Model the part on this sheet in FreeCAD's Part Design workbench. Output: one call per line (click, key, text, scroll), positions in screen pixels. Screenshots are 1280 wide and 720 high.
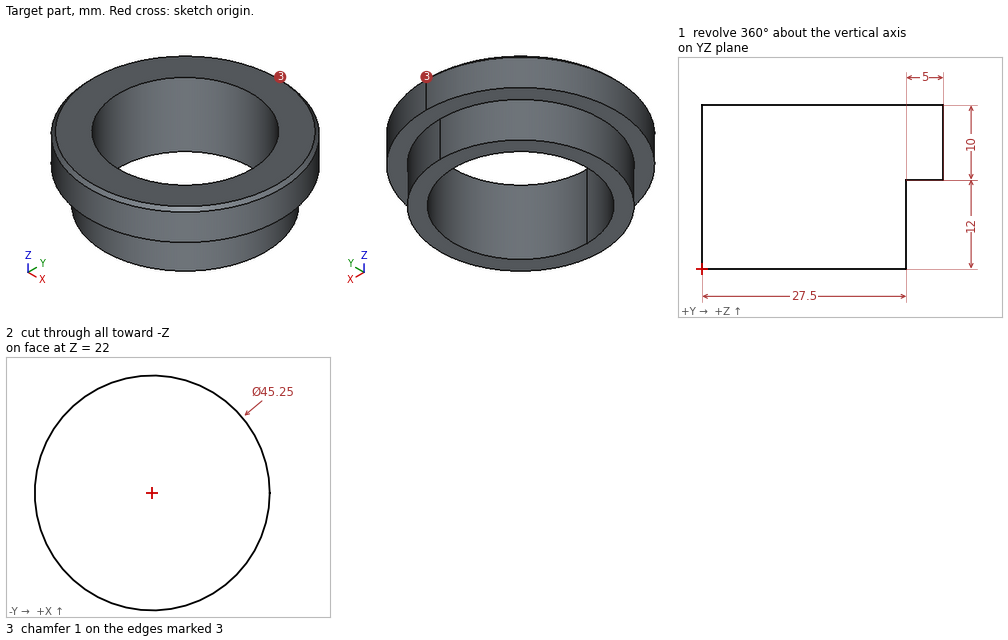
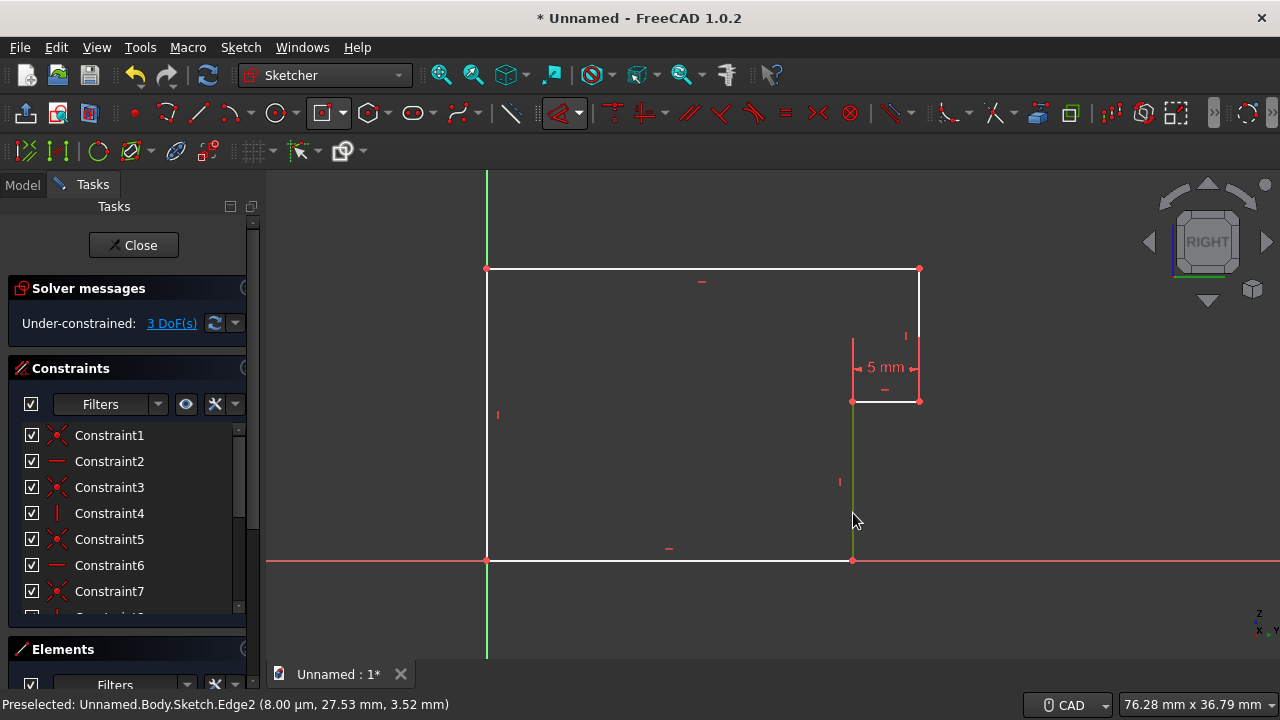
key(i)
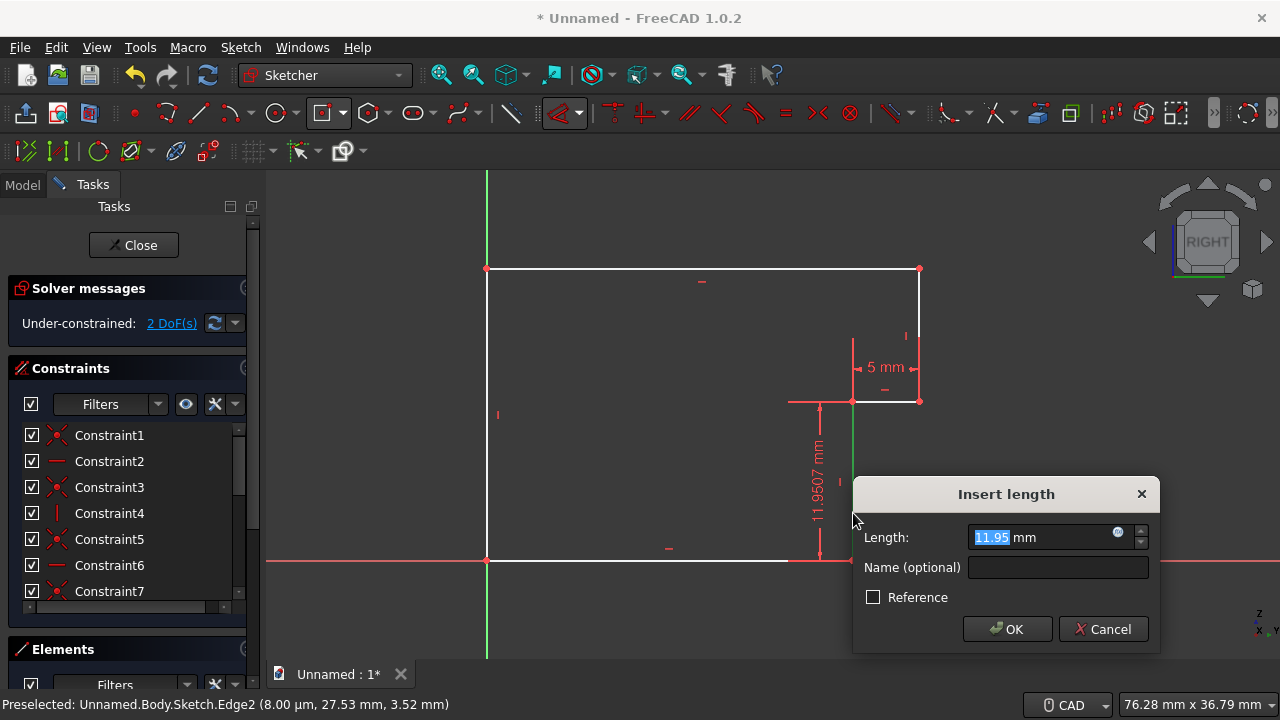
text(12)
key(Return)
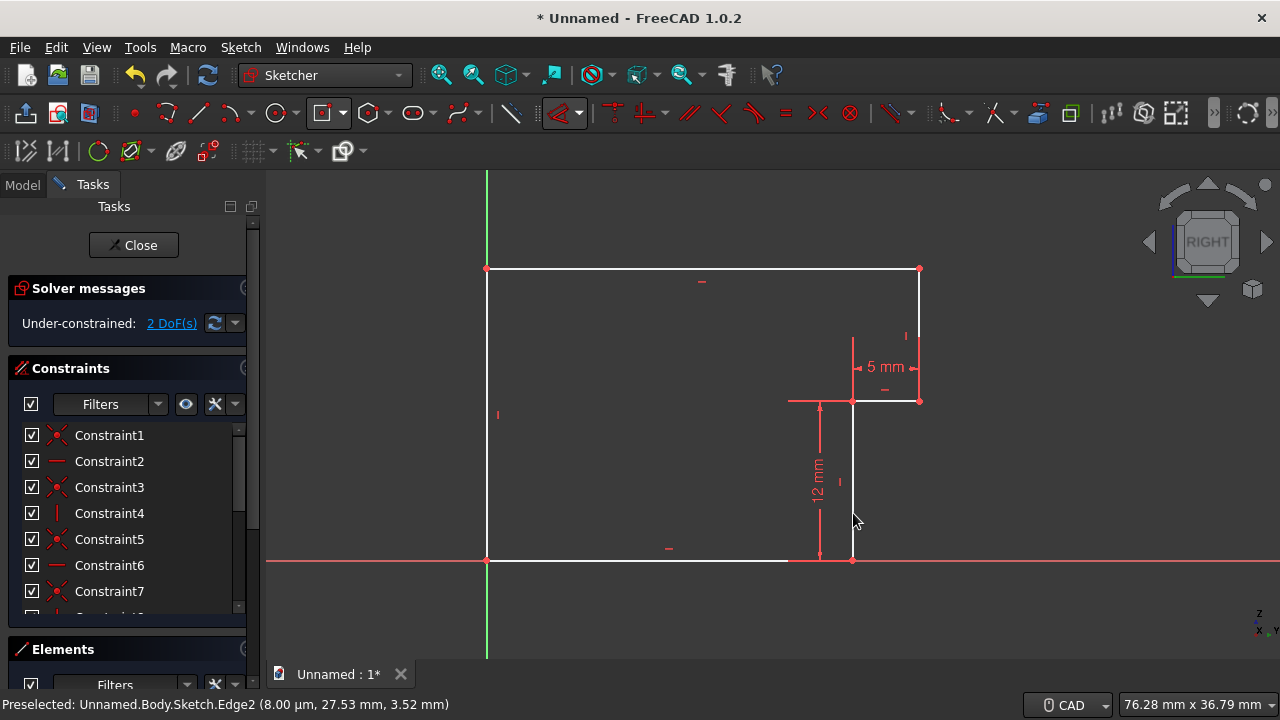
click(919, 362)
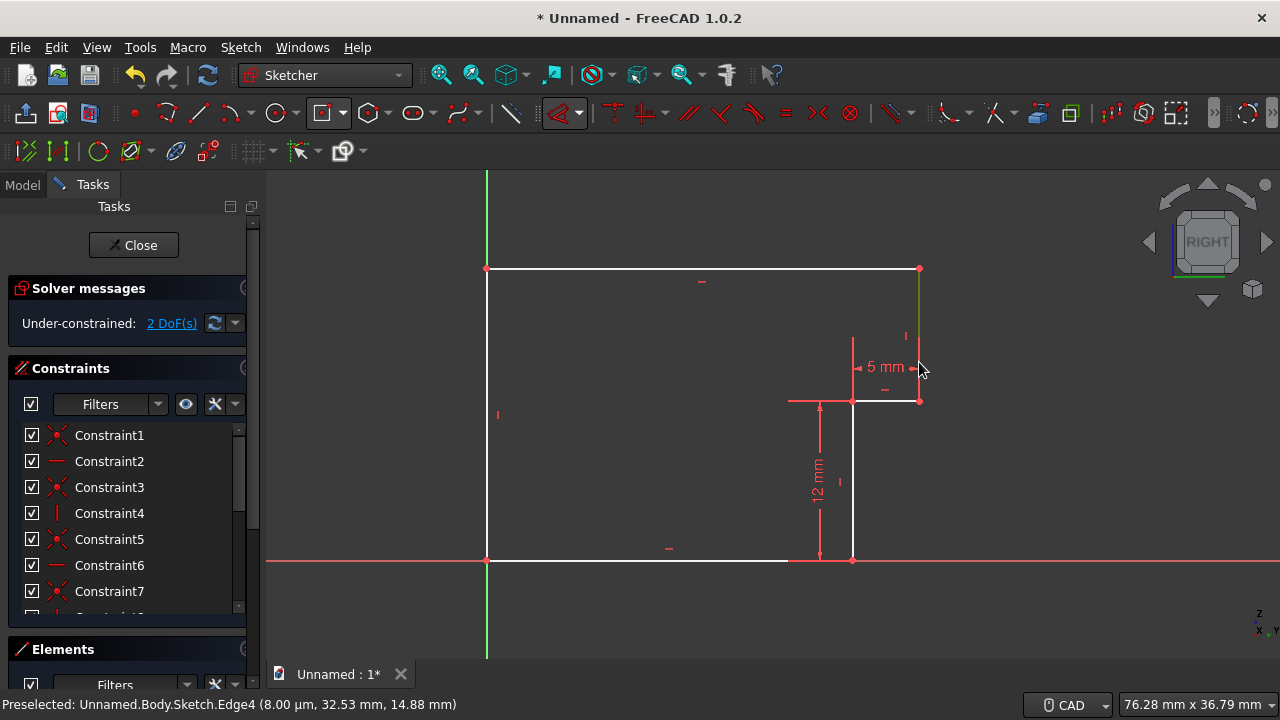
click(582, 114)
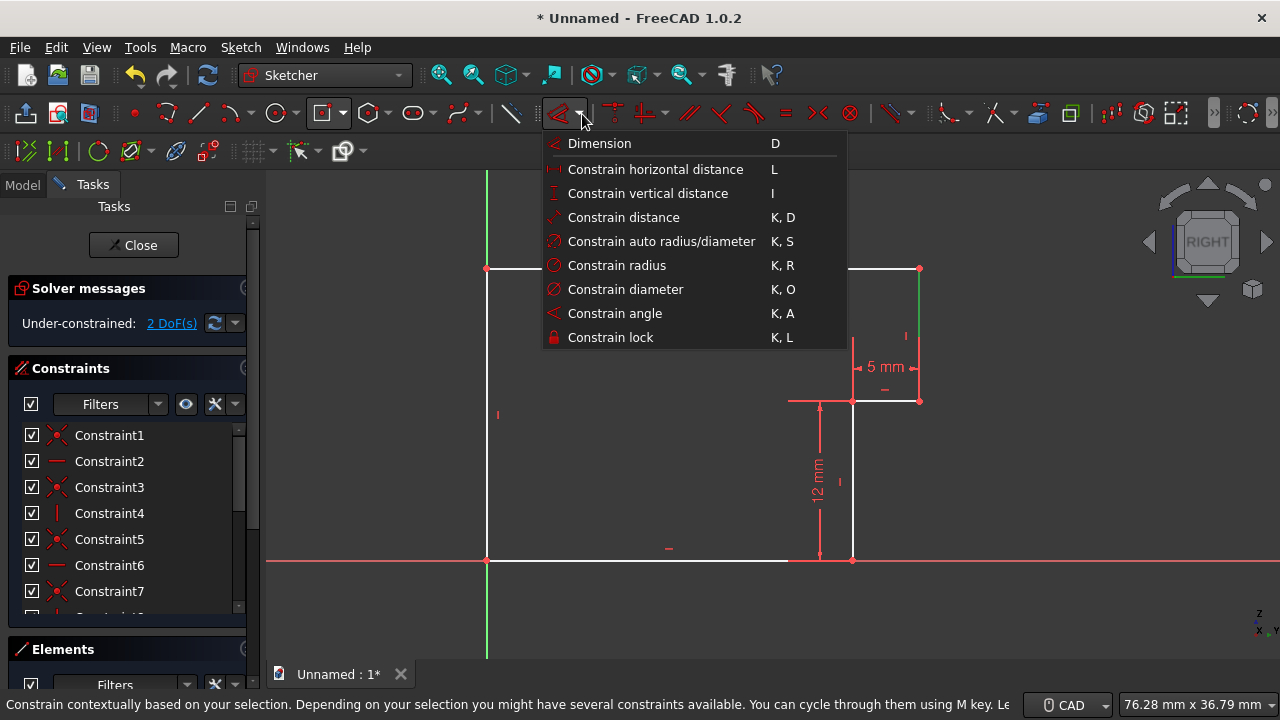
click(695, 193)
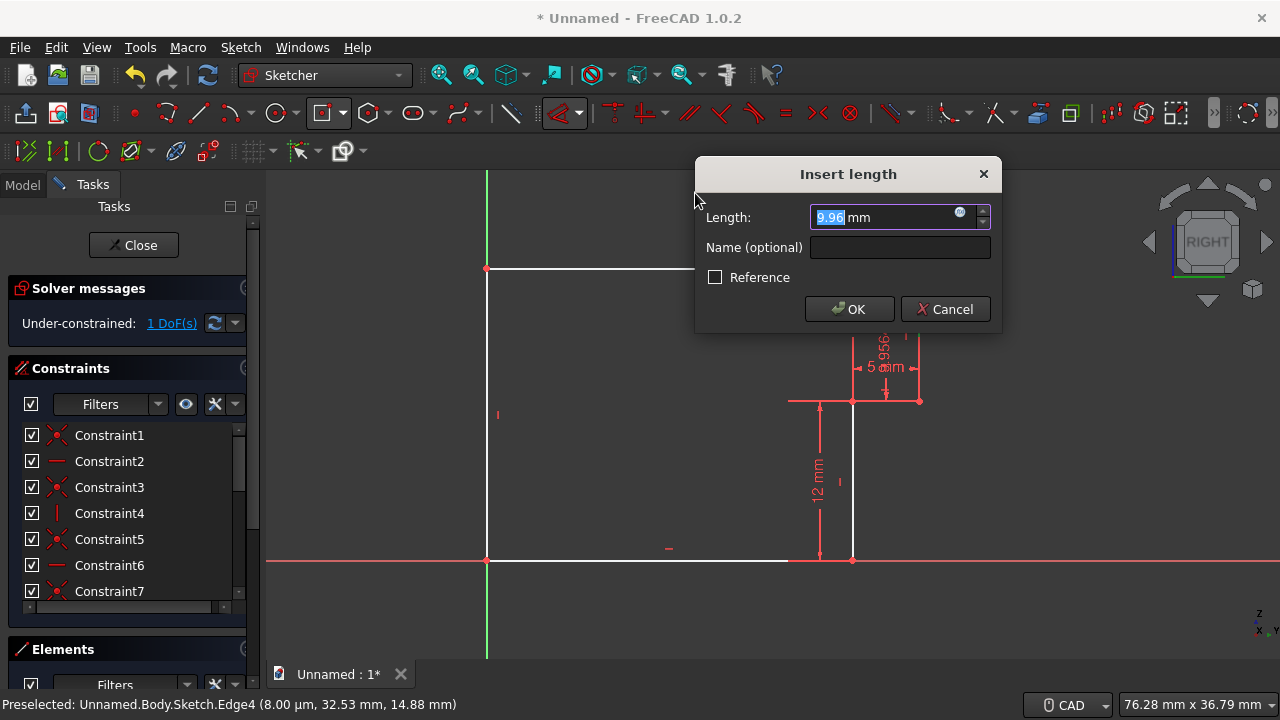
text(10)
key(Return)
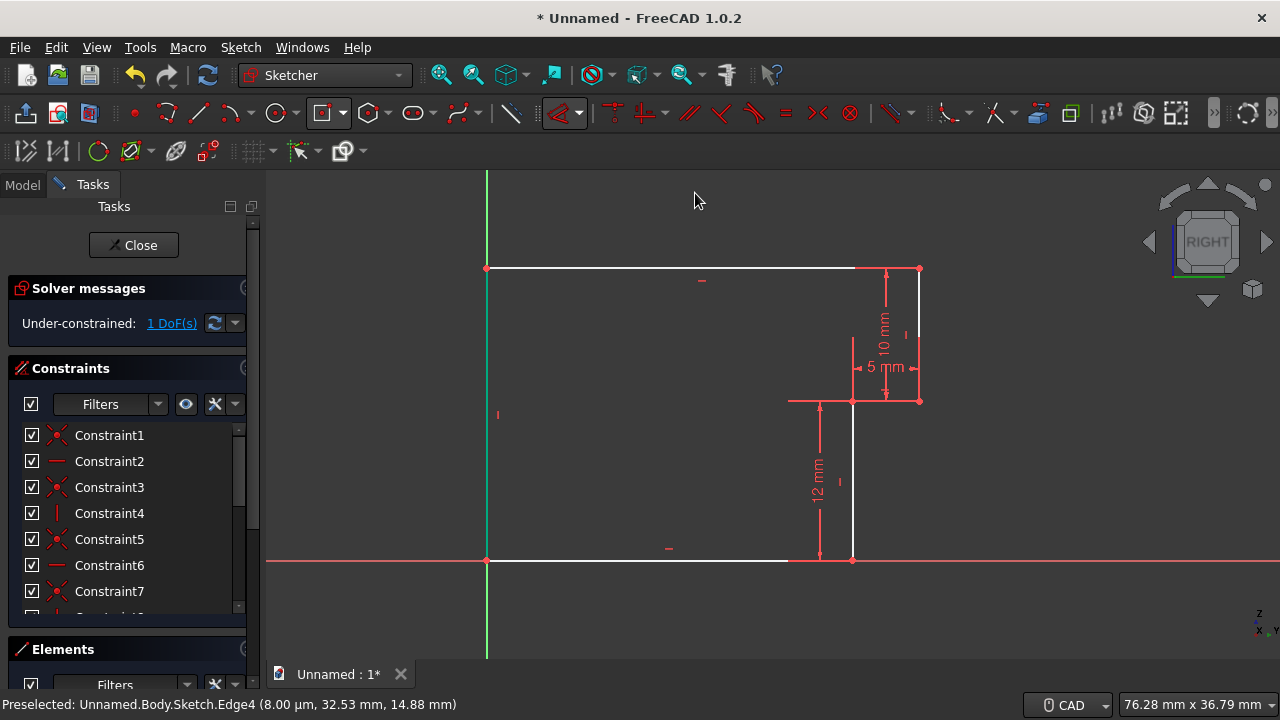
click(596, 561)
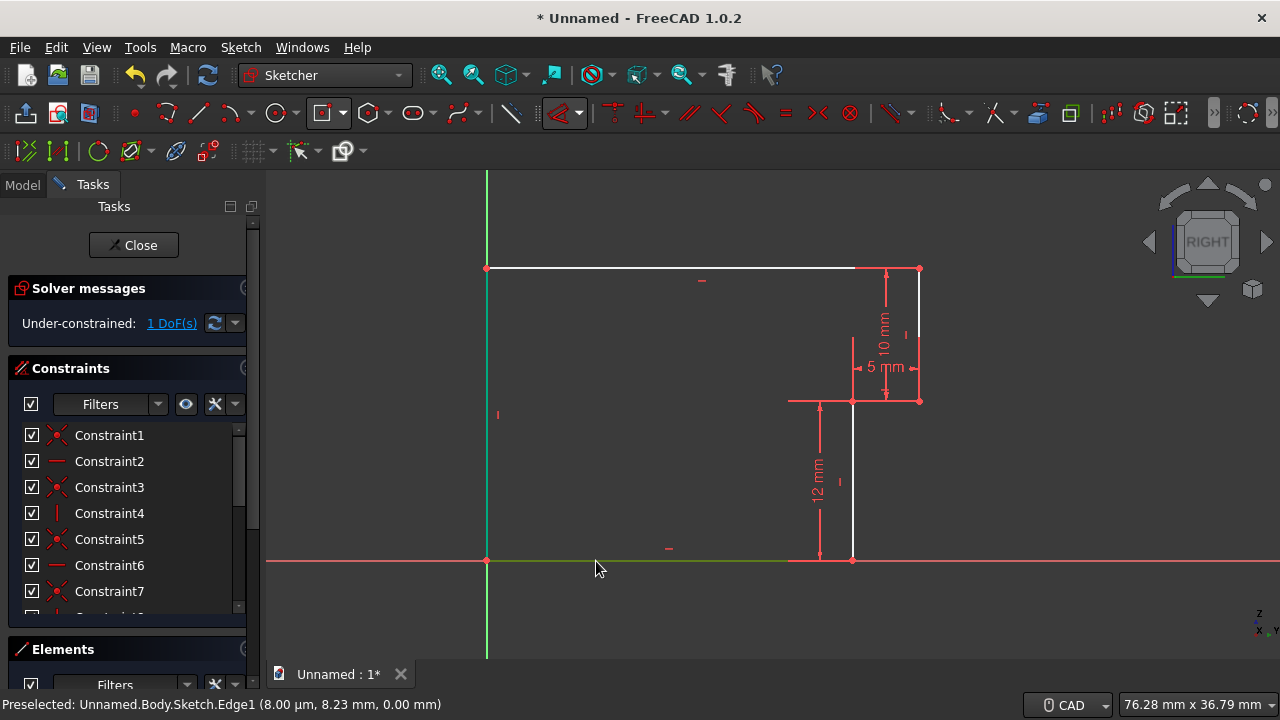
key(l)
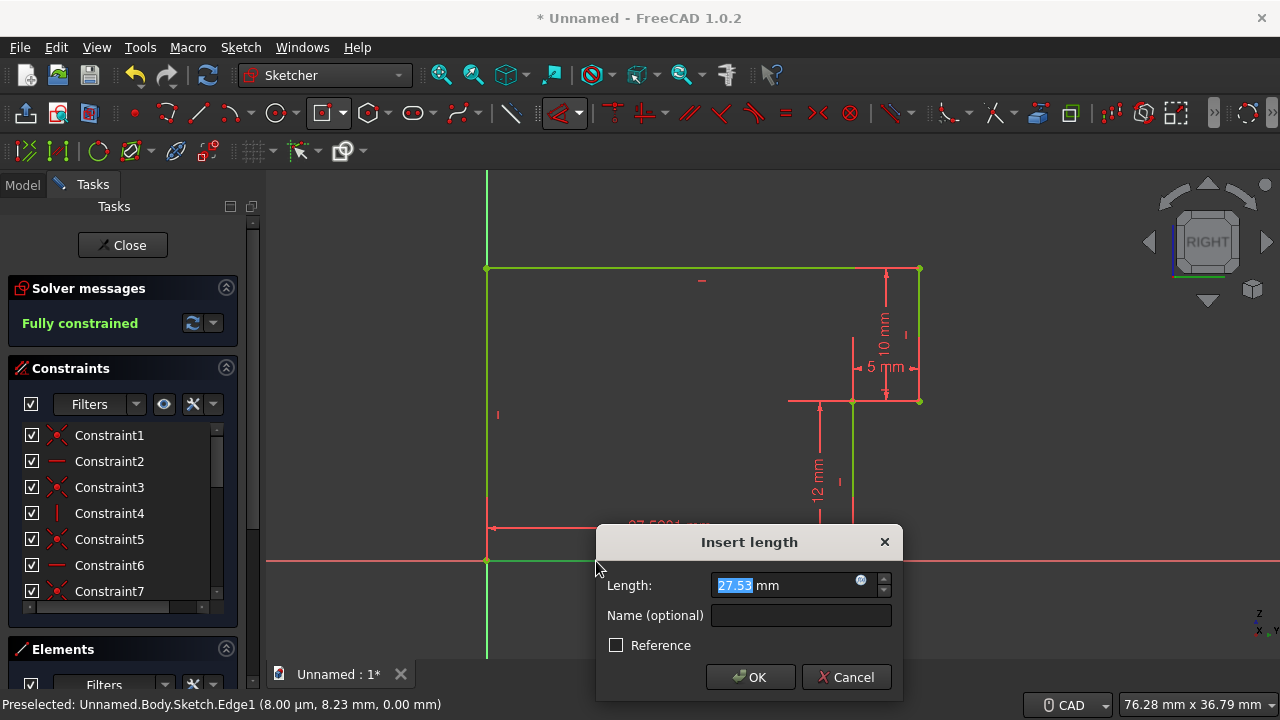
text(27.5)
key(Return)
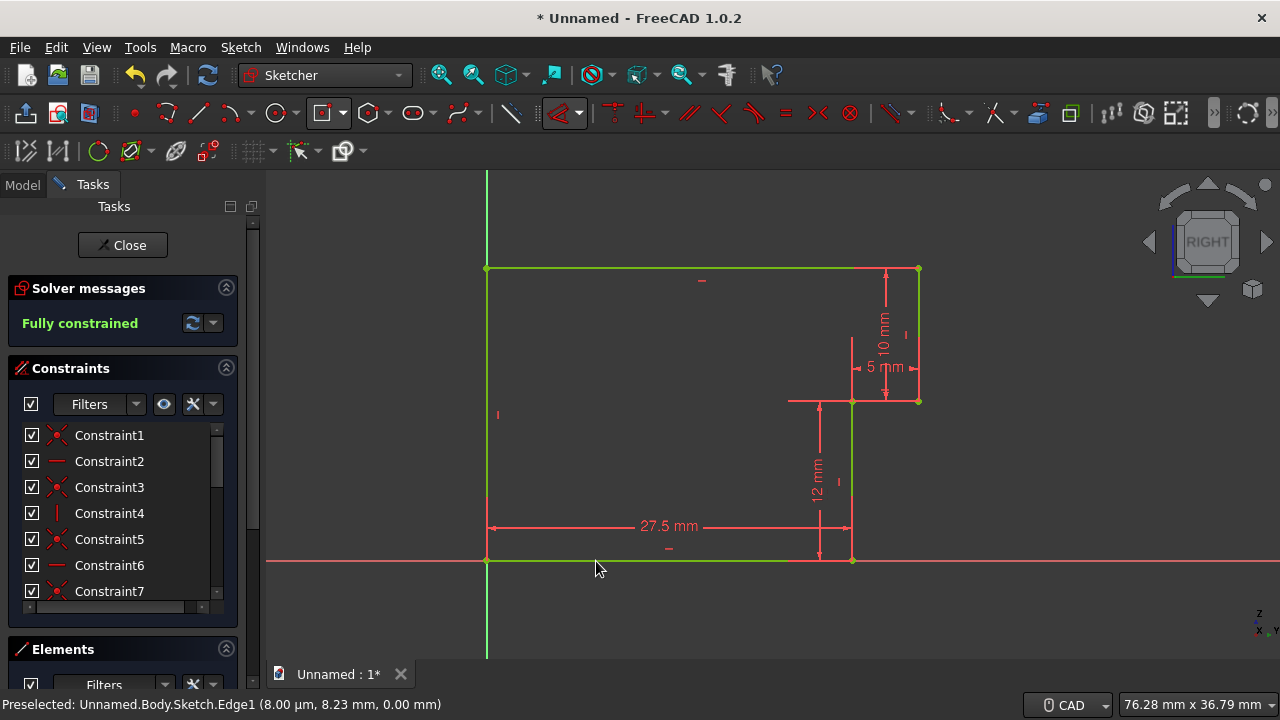
click(123, 245)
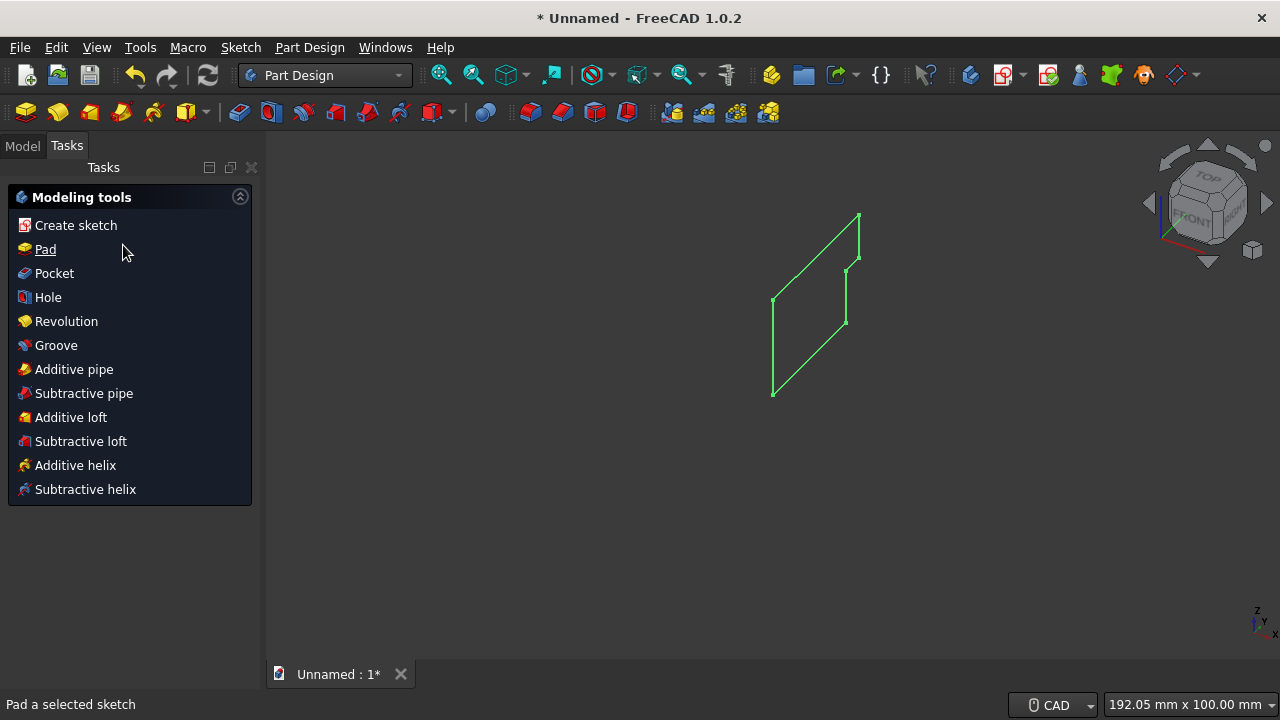
click(58, 112)